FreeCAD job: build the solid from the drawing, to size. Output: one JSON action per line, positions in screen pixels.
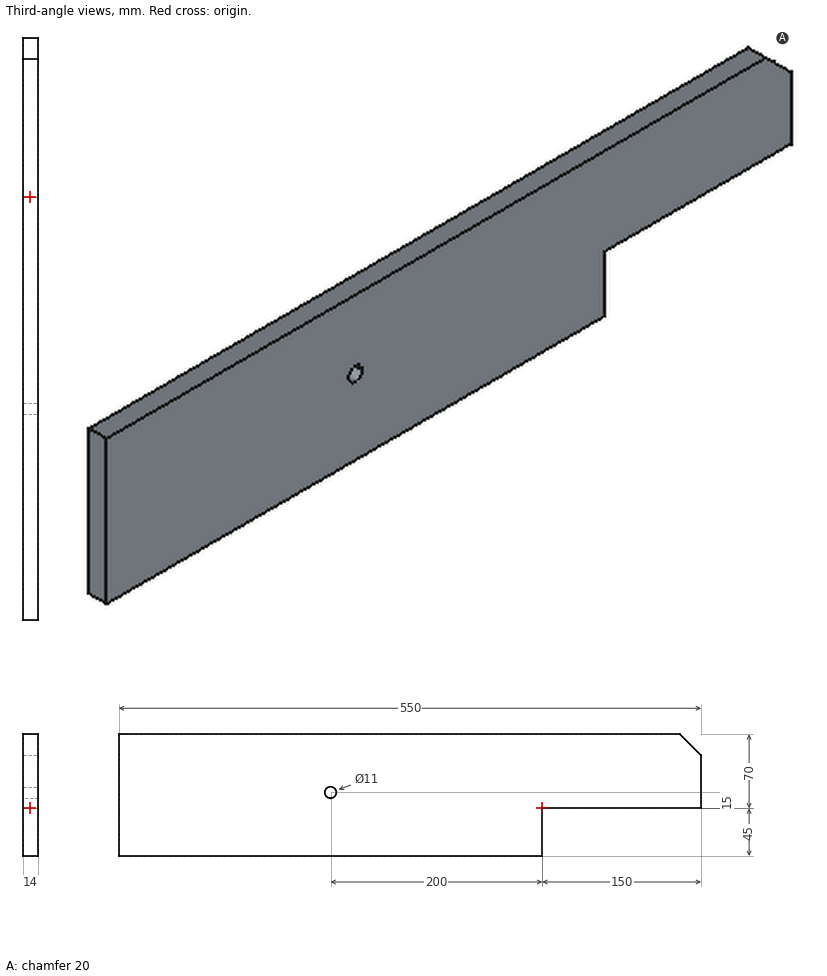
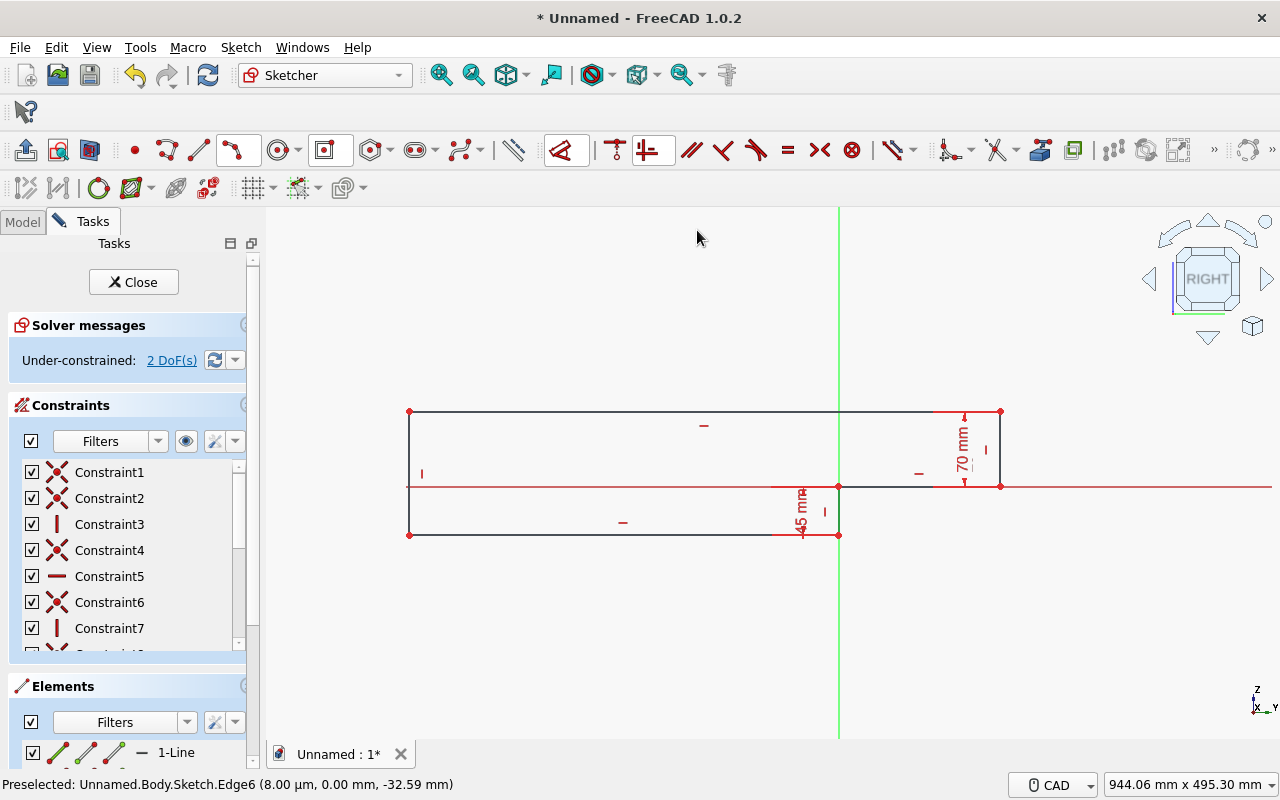
{"action": "left_click", "coordinate": [887, 487]}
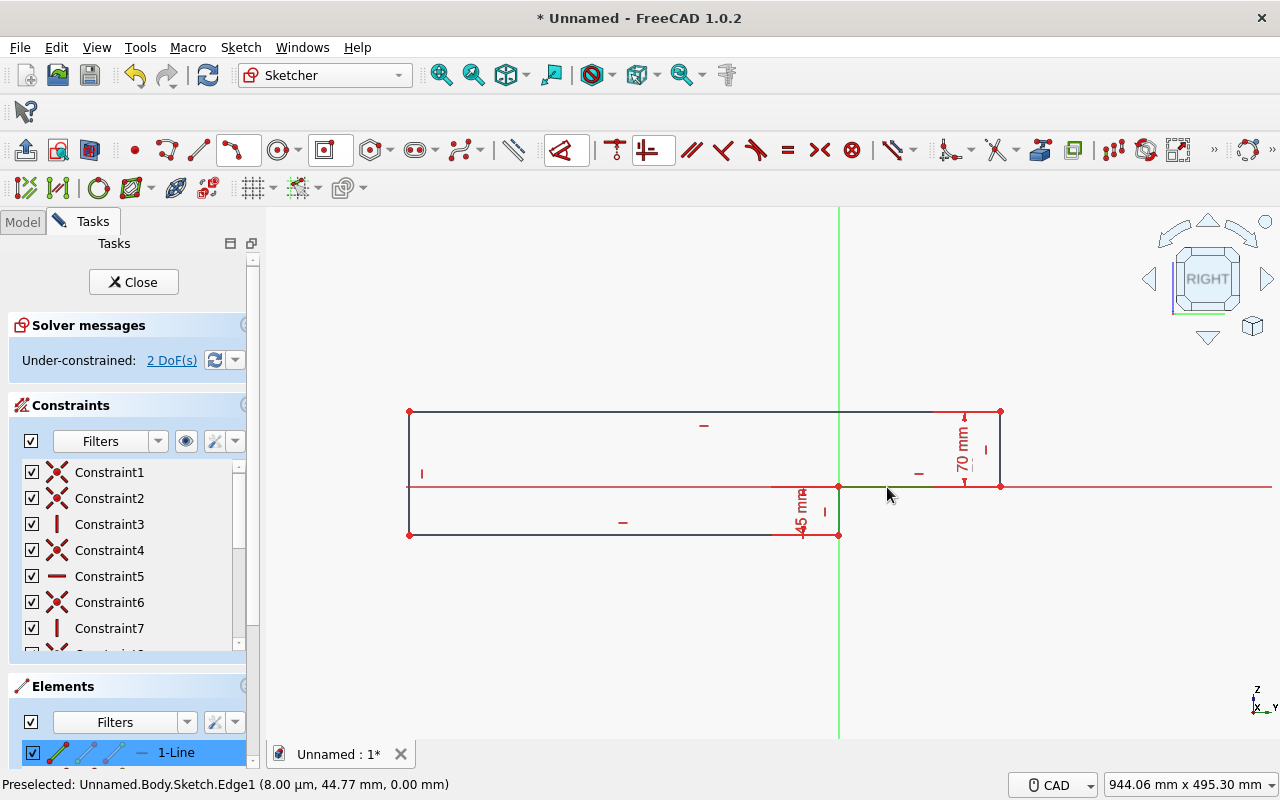
{"action": "key", "text": "l"}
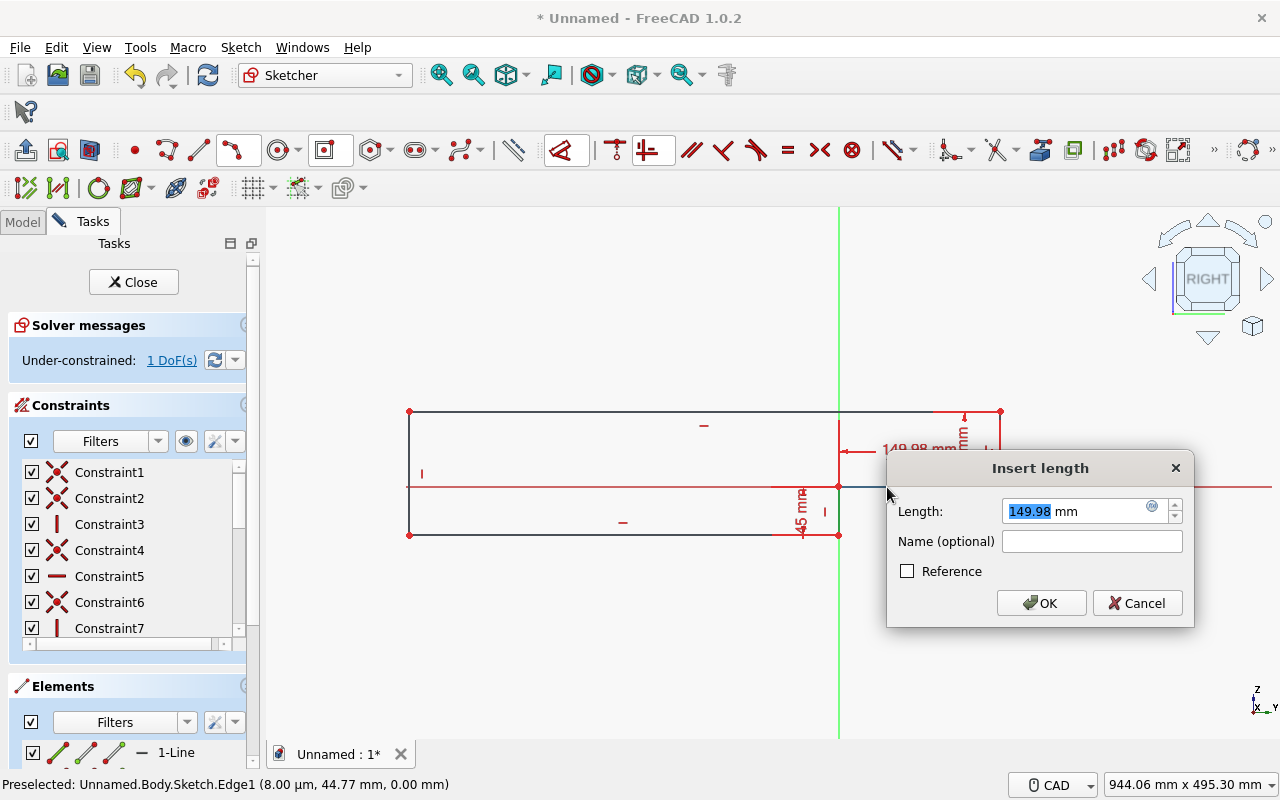
{"action": "type", "text": "150"}
{"action": "key", "text": "Return"}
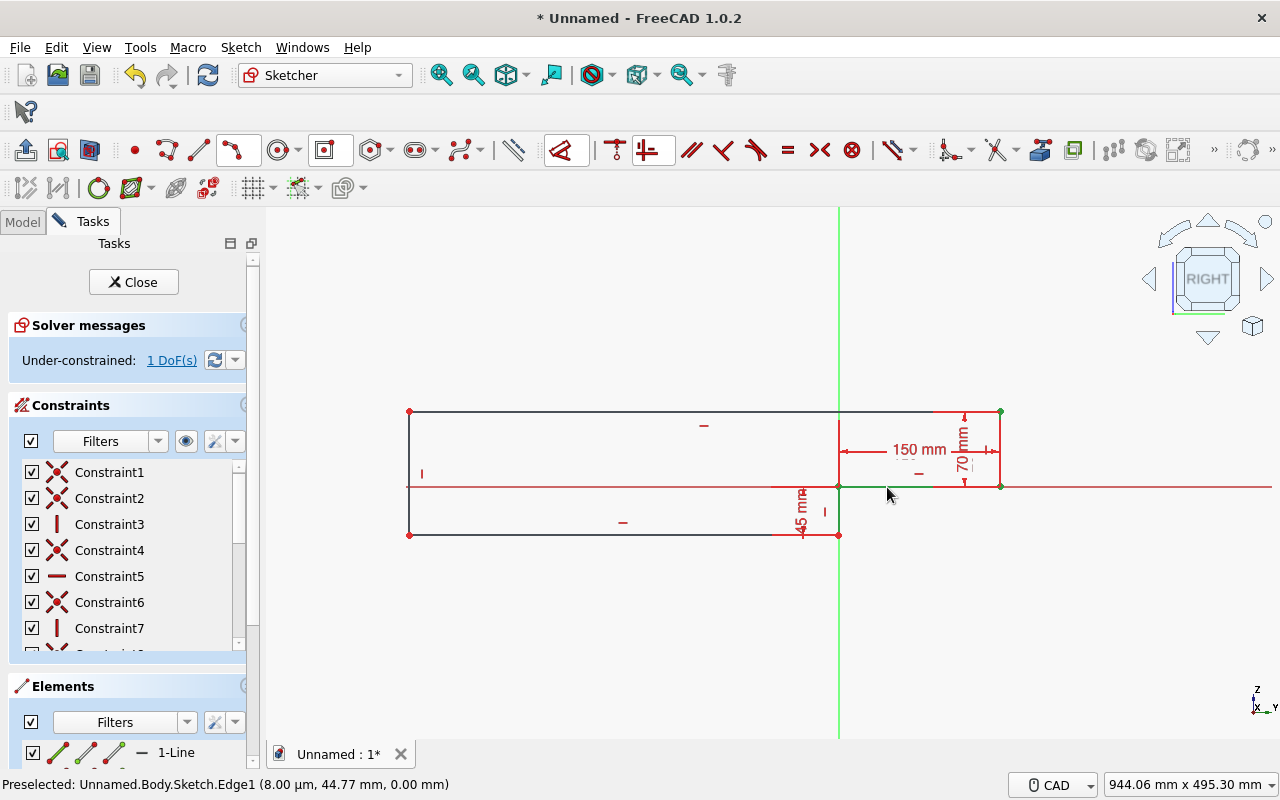
{"action": "left_click", "coordinate": [823, 412]}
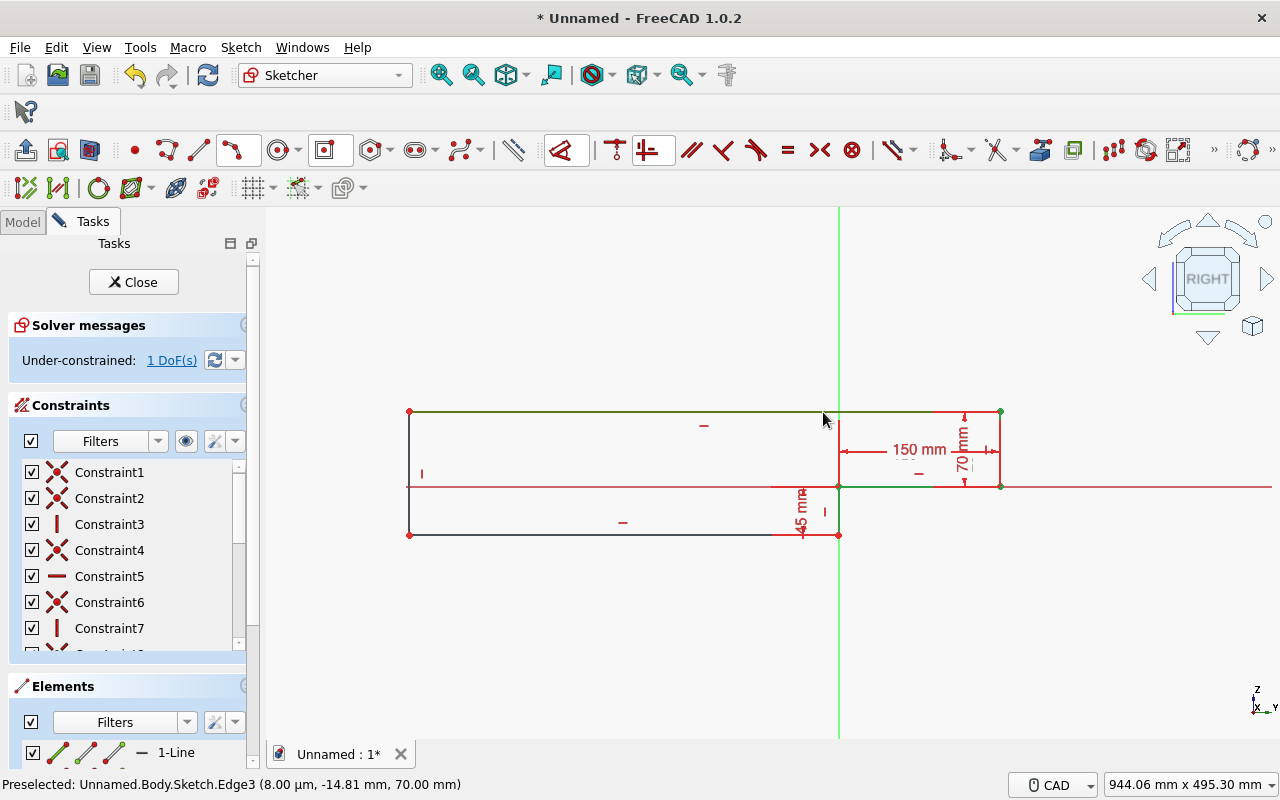
{"action": "left_click", "coordinate": [584, 150]}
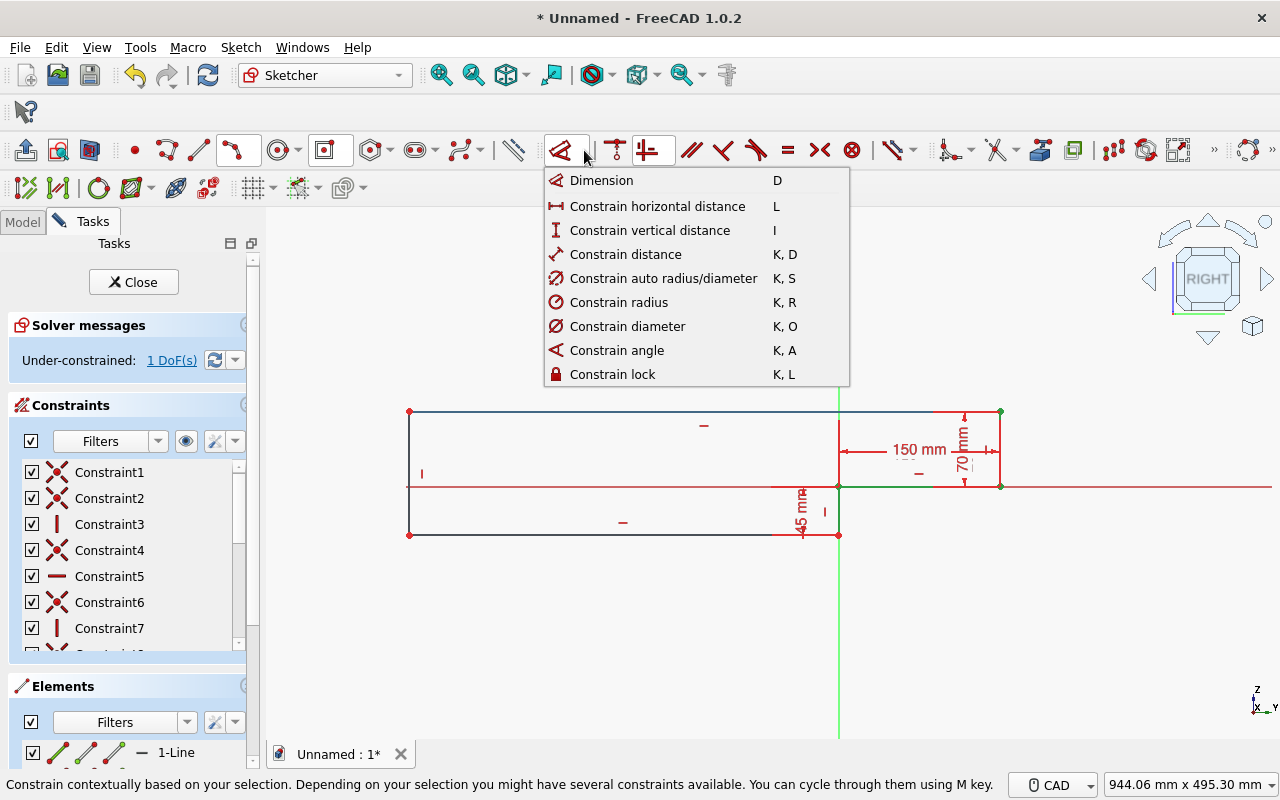
{"action": "left_click", "coordinate": [697, 206]}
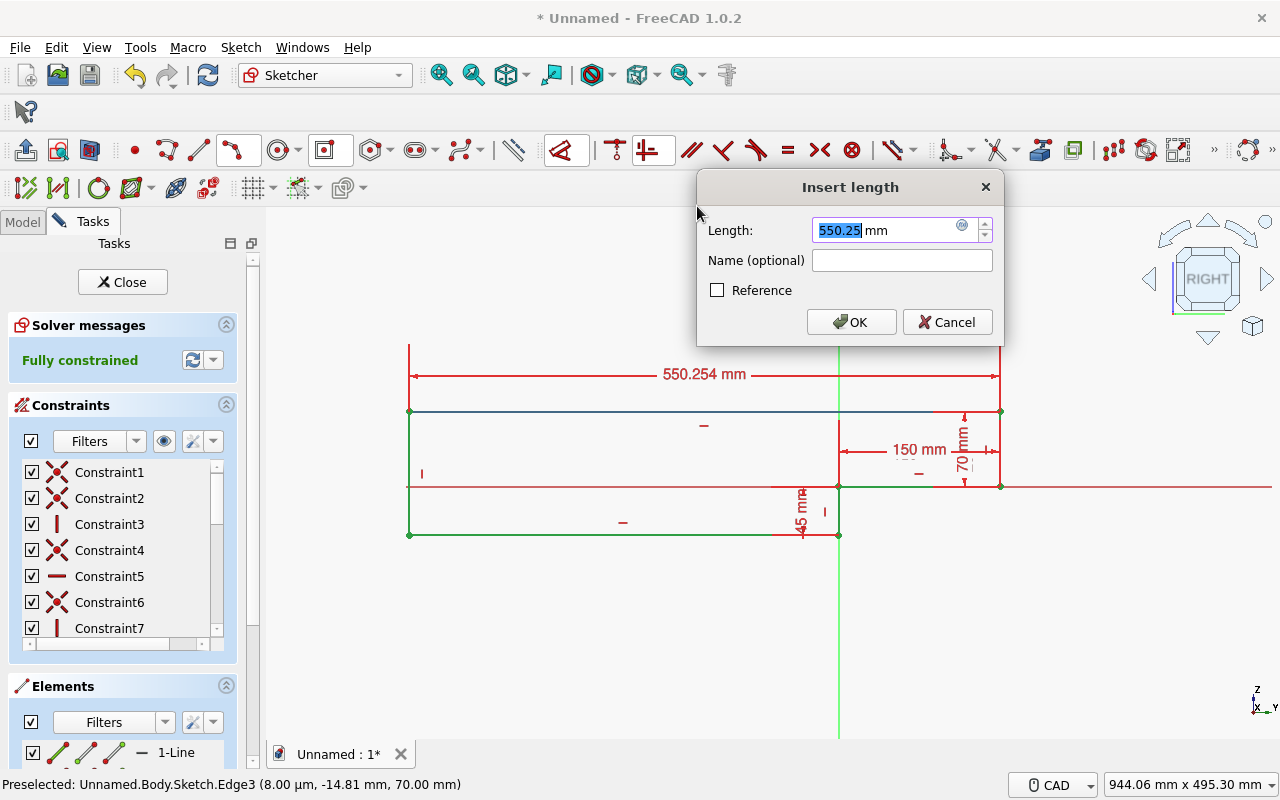
{"action": "type", "text": "550"}
{"action": "key", "text": "Return"}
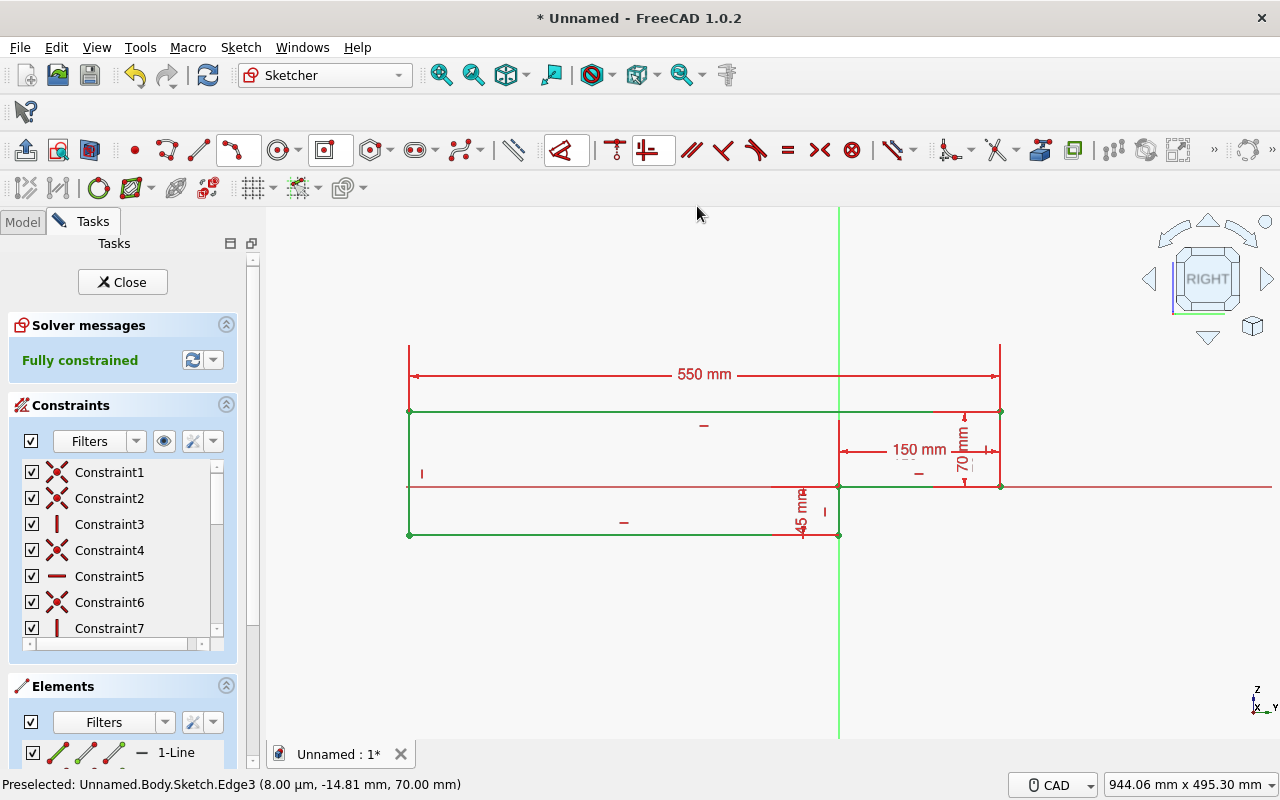
{"action": "left_click", "coordinate": [123, 282]}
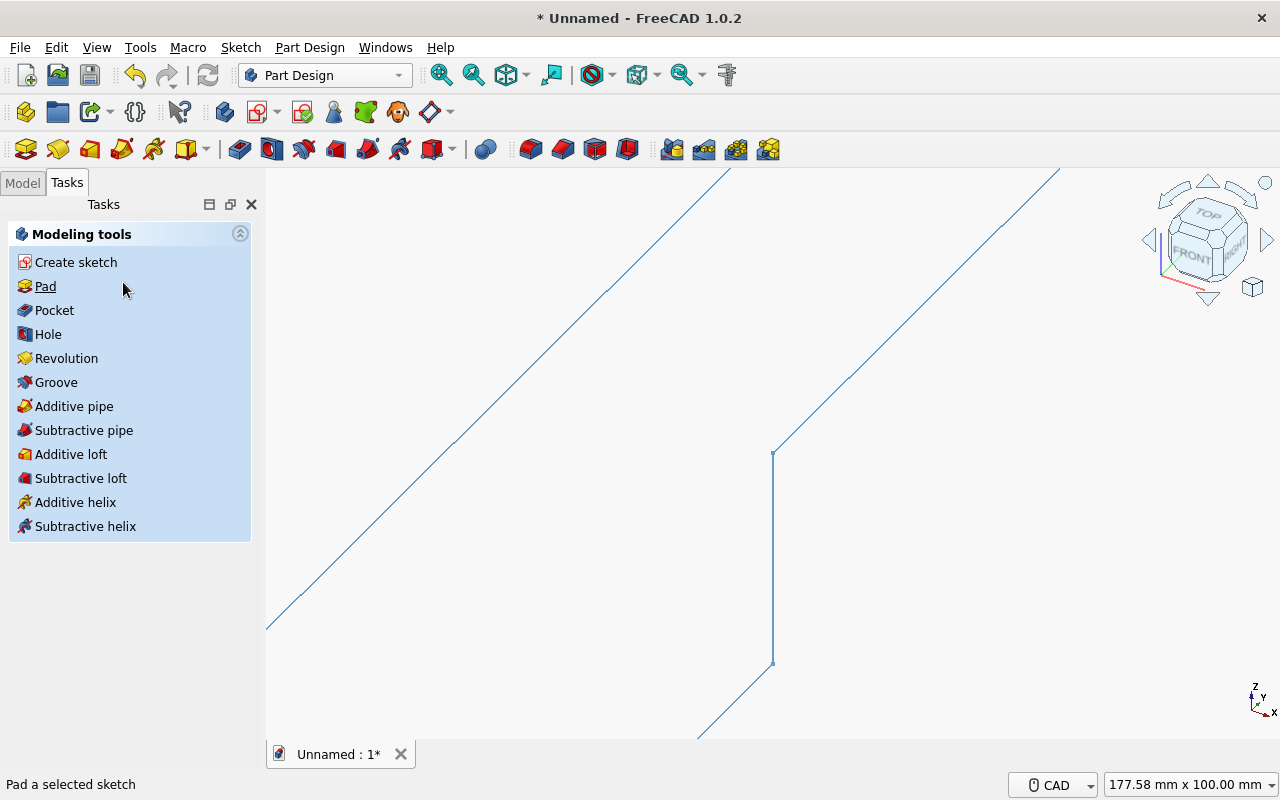
{"action": "left_click", "coordinate": [26, 150]}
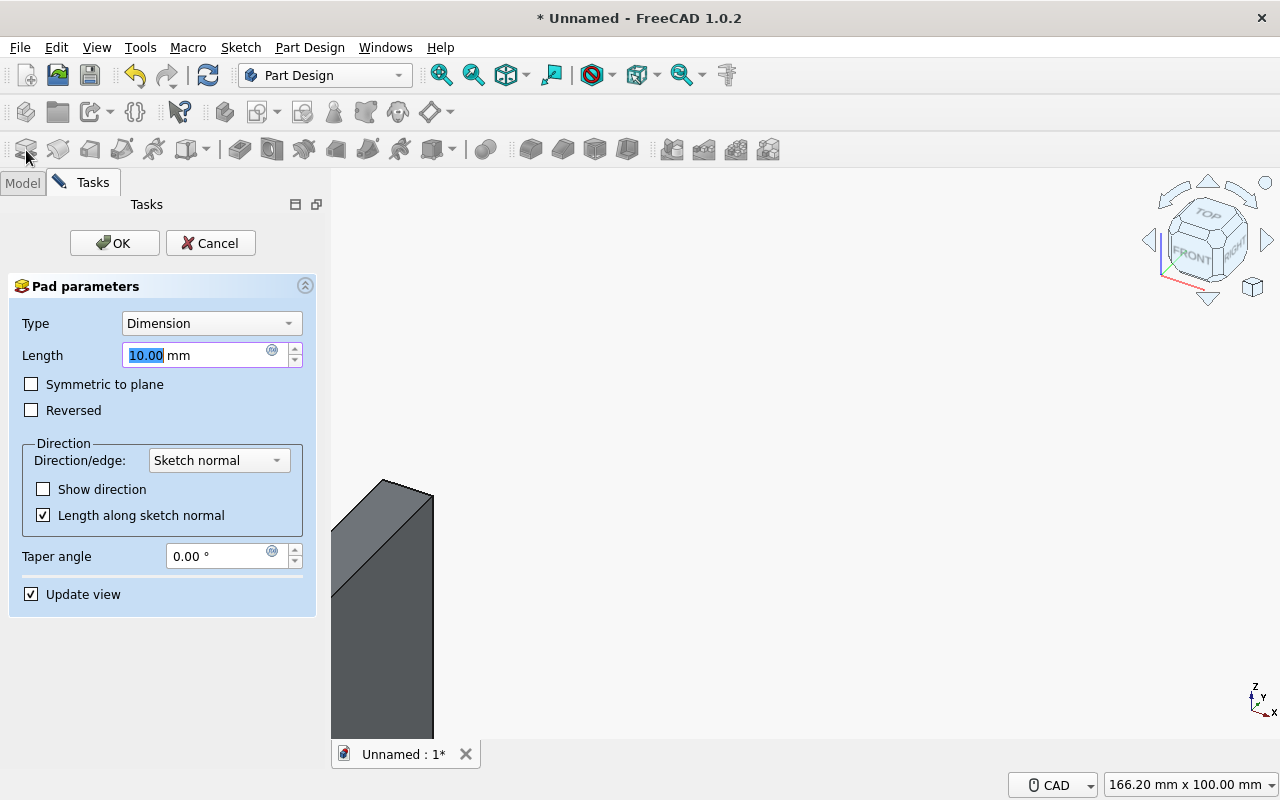
{"action": "type", "text": "14"}
{"action": "key", "text": "Tab"}